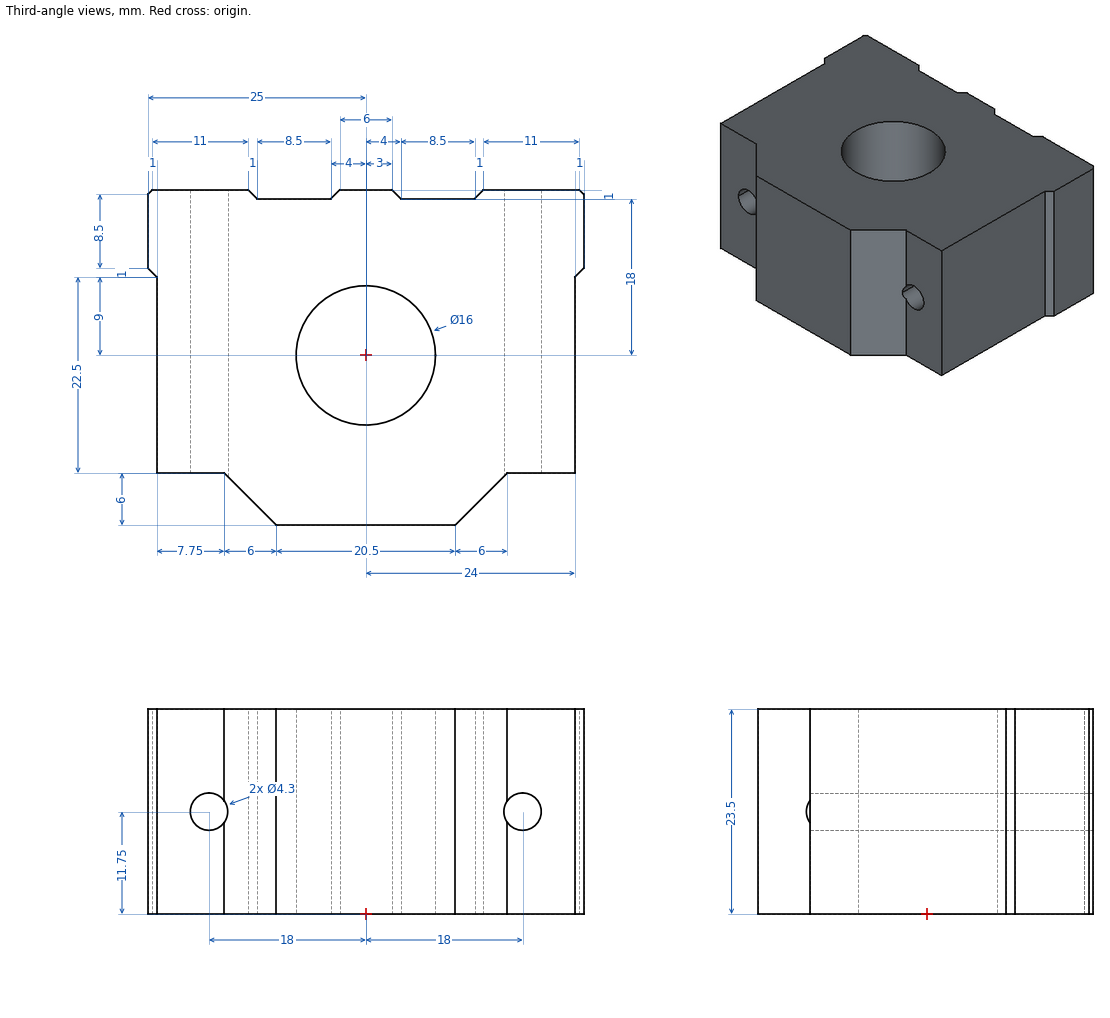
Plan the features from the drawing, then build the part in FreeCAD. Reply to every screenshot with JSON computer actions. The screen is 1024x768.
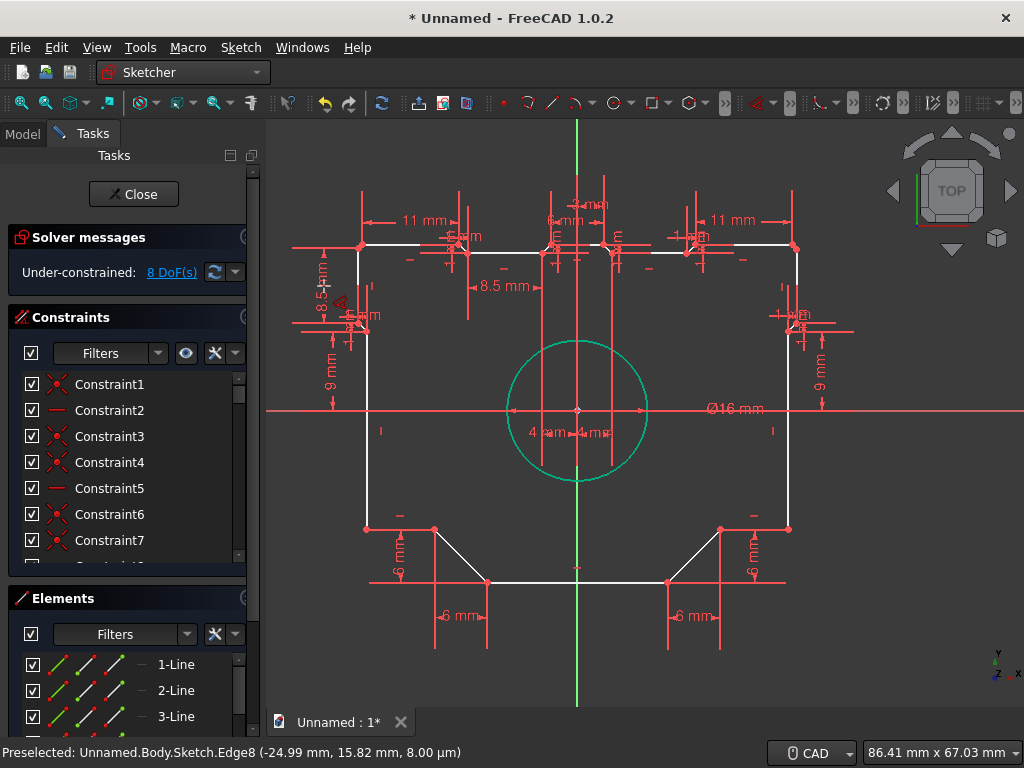
{"action": "left_click", "coordinate": [797, 301]}
{"action": "left_click", "coordinate": [831, 286]}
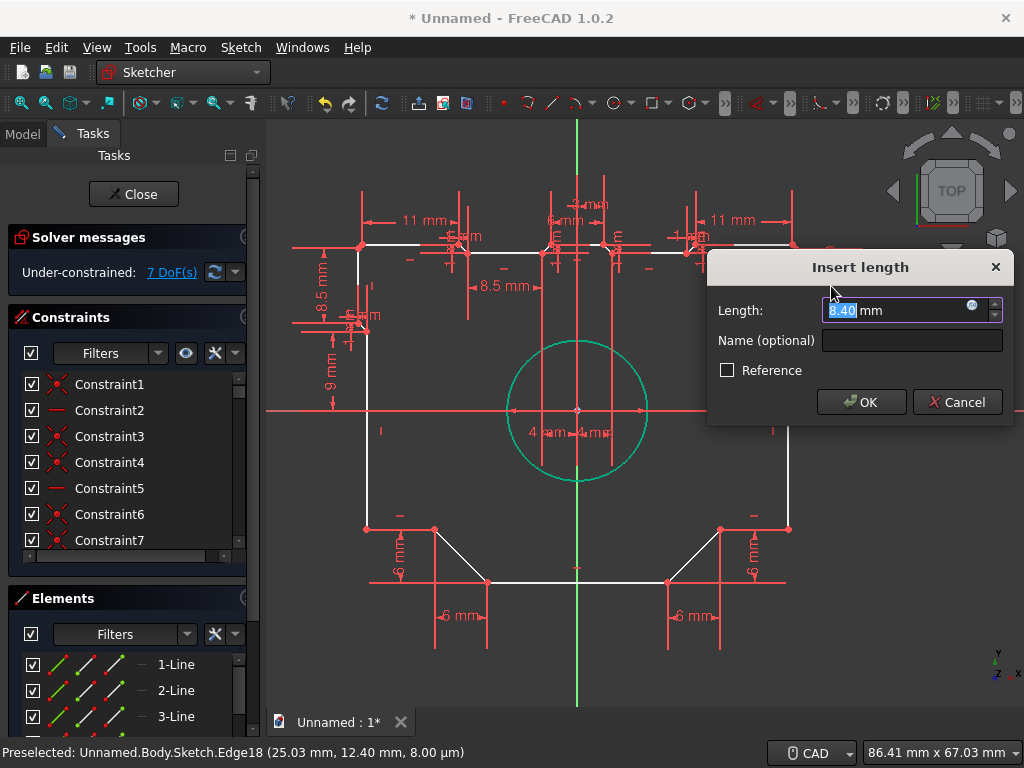
{"action": "type", "text": "8.5"}
{"action": "key", "text": "Return"}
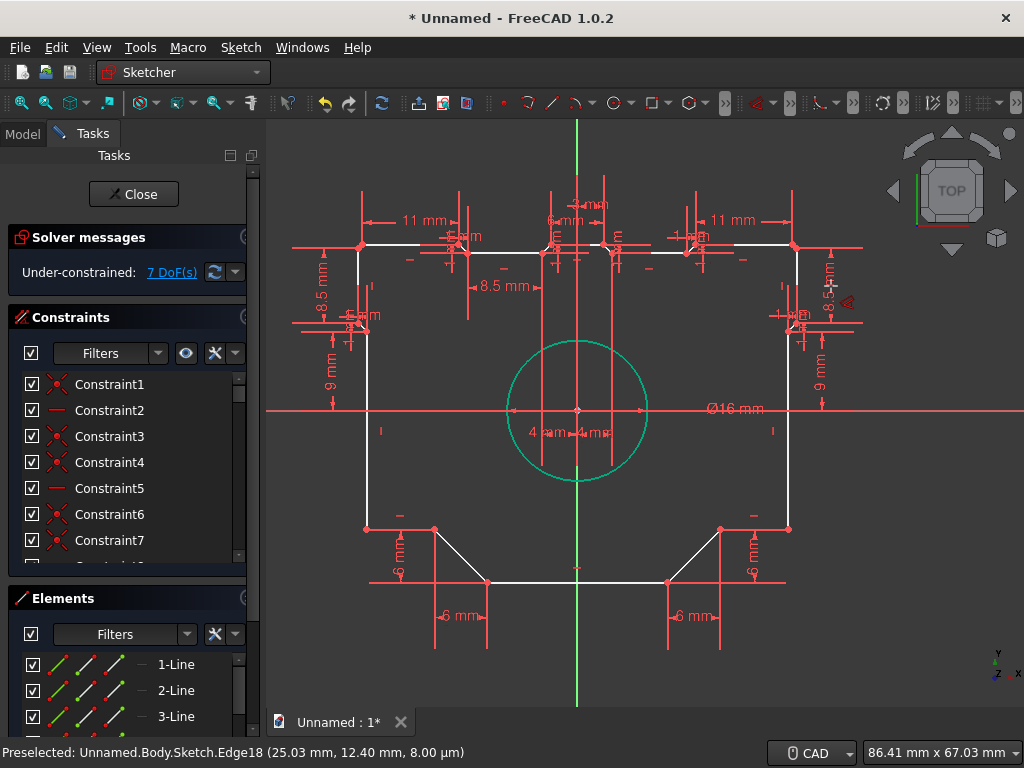
{"action": "left_click", "coordinate": [664, 253]}
{"action": "left_click", "coordinate": [650, 287]}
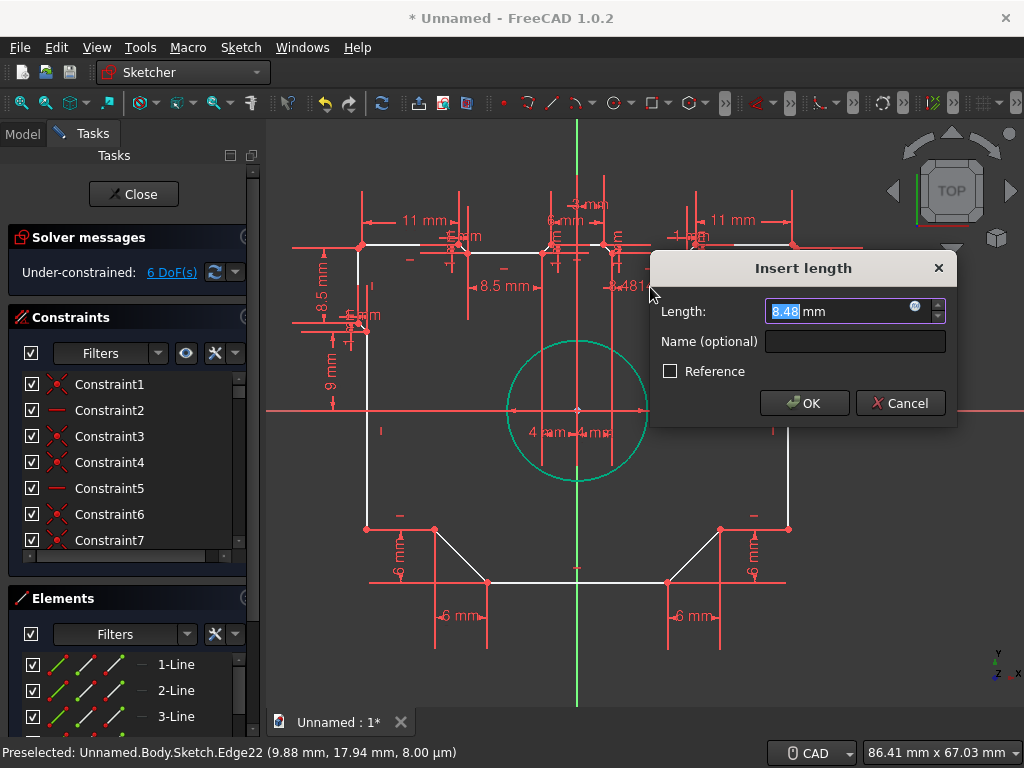
{"action": "type", "text": "8.5"}
{"action": "key", "text": "Return"}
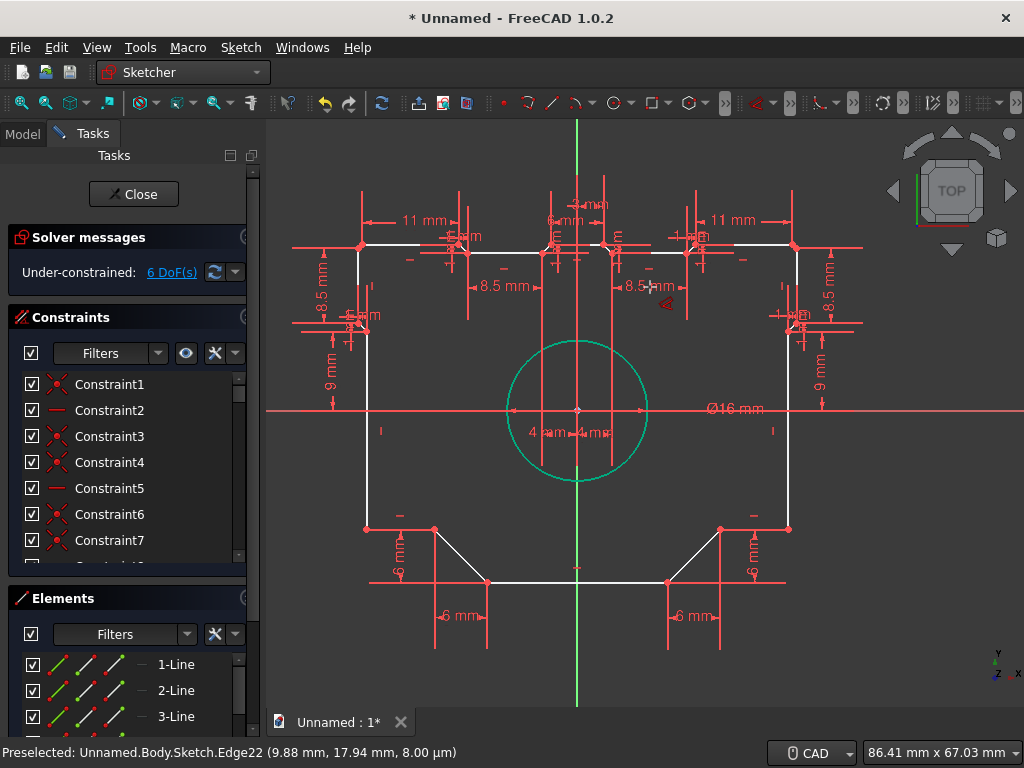
{"action": "left_click", "coordinate": [612, 253]}
{"action": "left_click", "coordinate": [646, 332]}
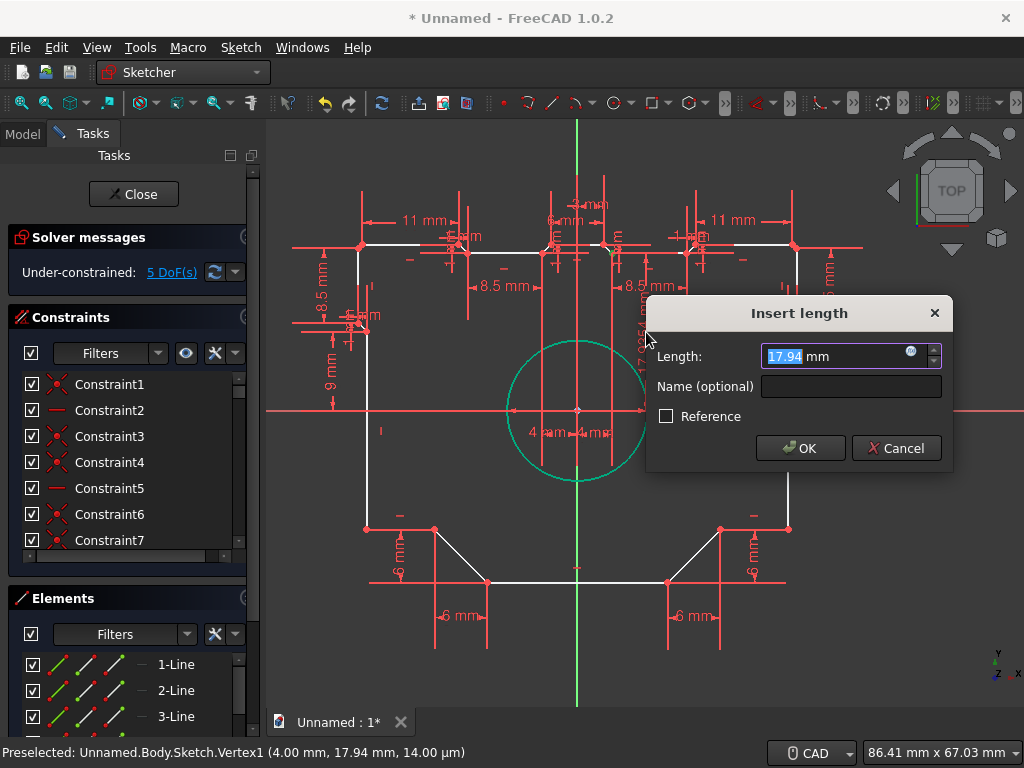
{"action": "type", "text": "18"}
{"action": "key", "text": "Return"}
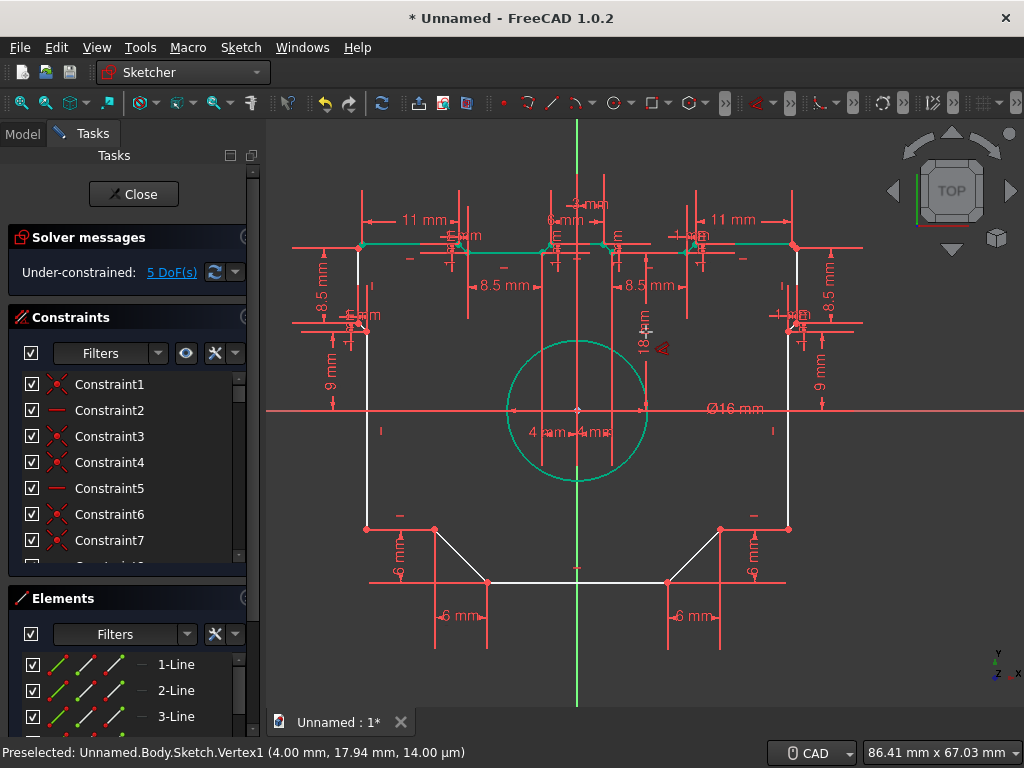
{"action": "scroll", "coordinate": [358, 248], "scroll_direction": "up", "scroll_amount": 4}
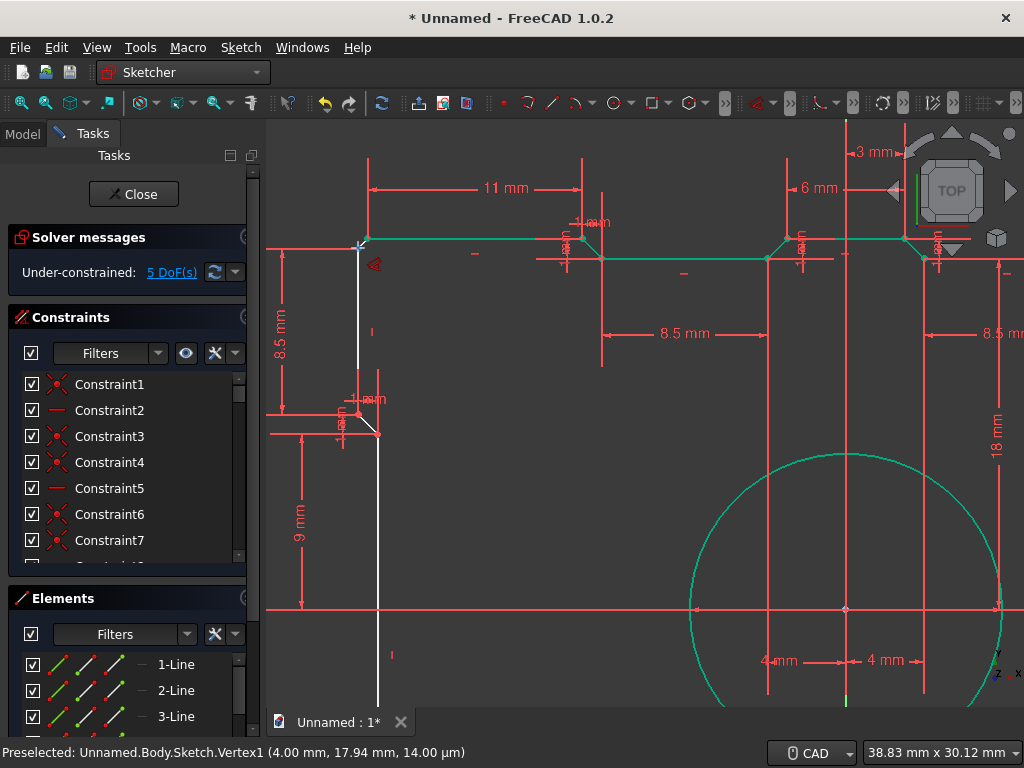
{"action": "left_click", "coordinate": [358, 249]}
{"action": "left_click", "coordinate": [490, 215]}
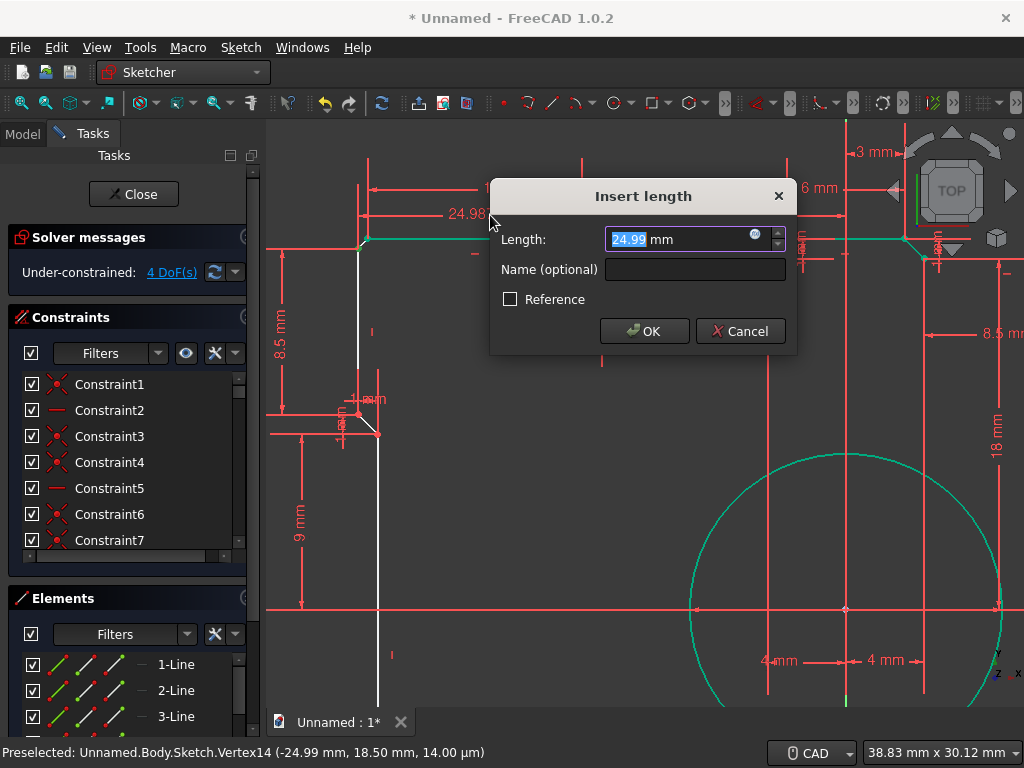
{"action": "type", "text": "25"}
{"action": "key", "text": "Return"}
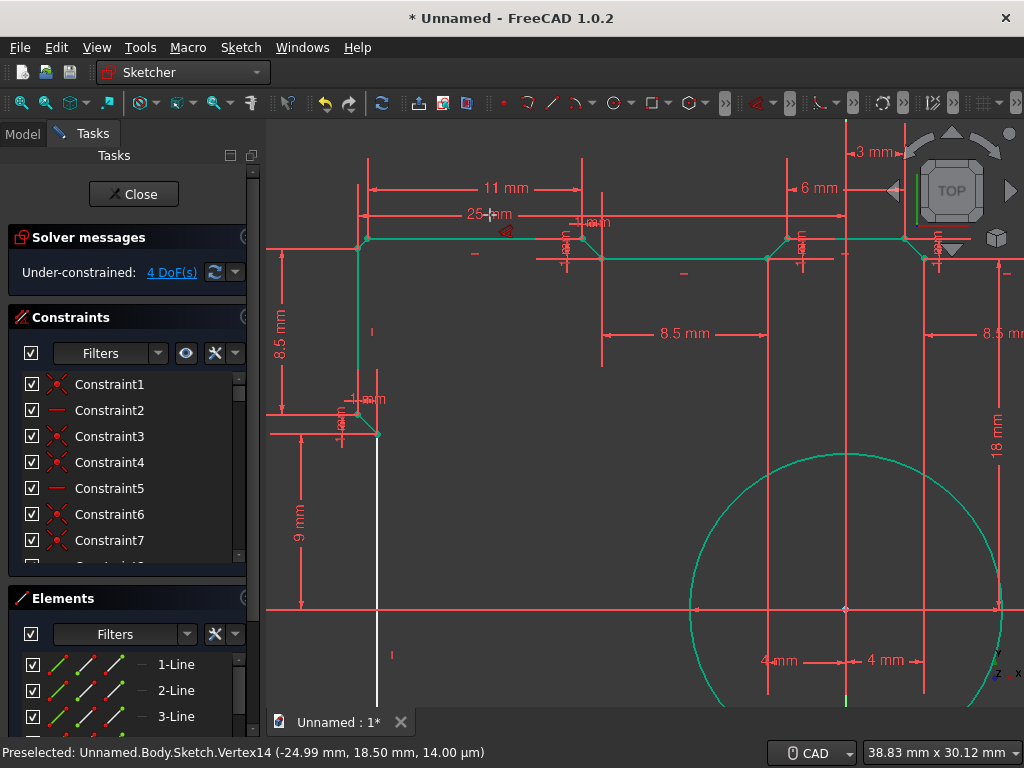
{"action": "scroll", "coordinate": [357, 248], "scroll_direction": "down", "scroll_amount": 4}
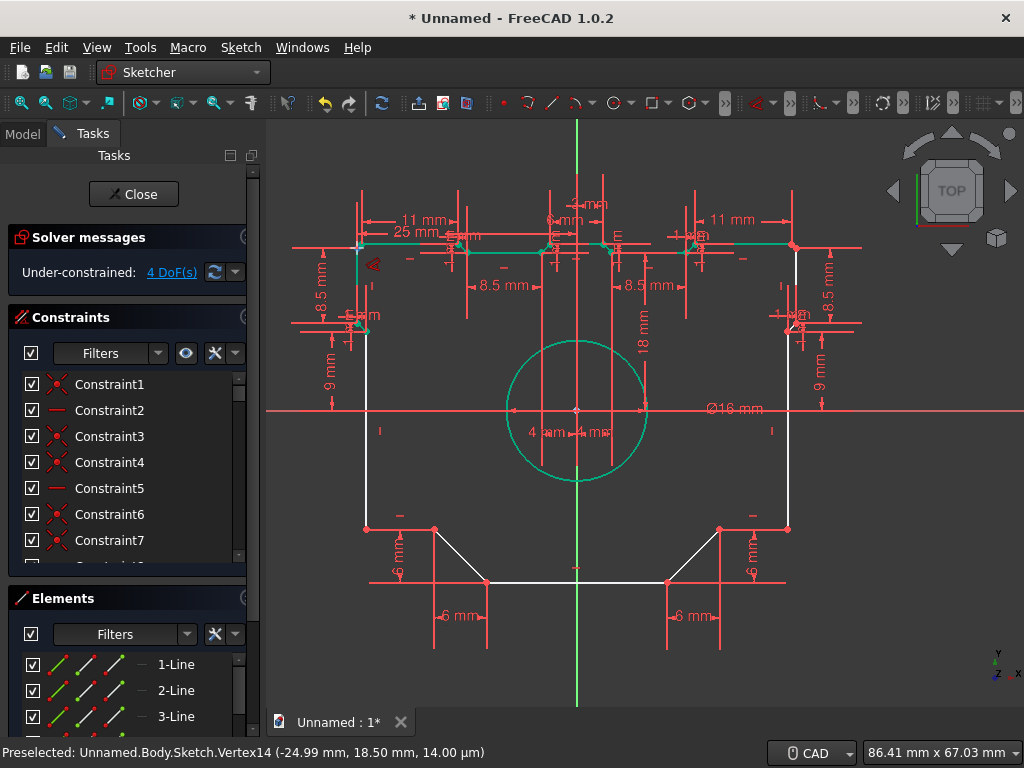
{"action": "left_click", "coordinate": [788, 530]}
{"action": "left_click", "coordinate": [634, 564]}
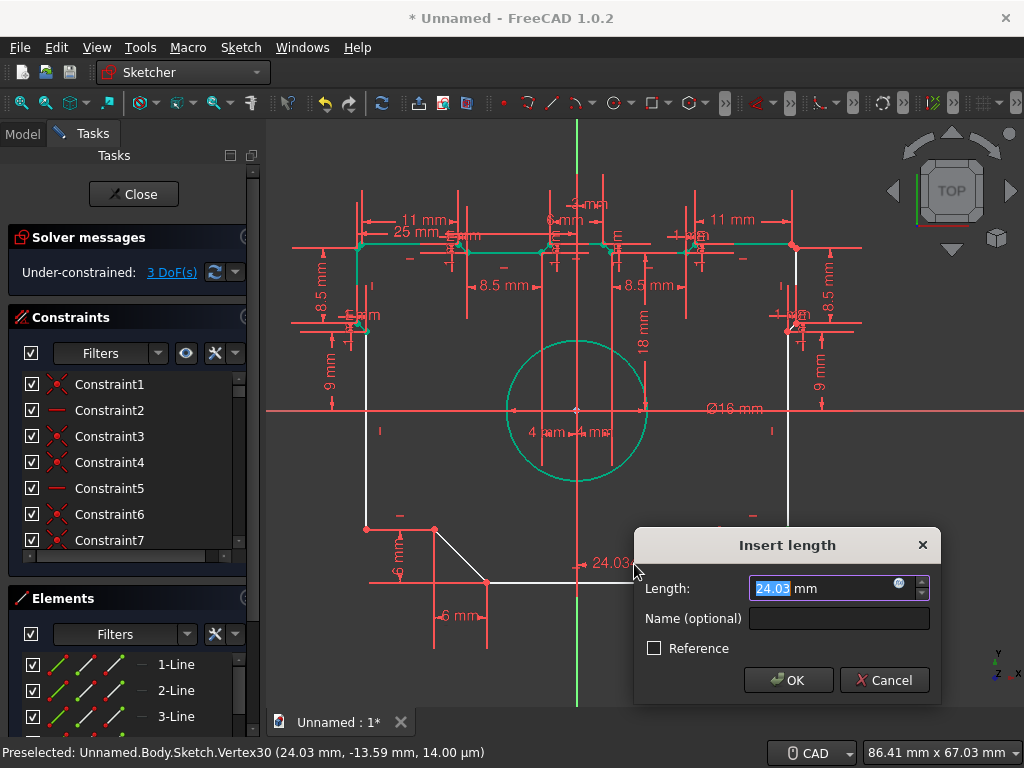
{"action": "type", "text": "24"}
{"action": "key", "text": "Return"}